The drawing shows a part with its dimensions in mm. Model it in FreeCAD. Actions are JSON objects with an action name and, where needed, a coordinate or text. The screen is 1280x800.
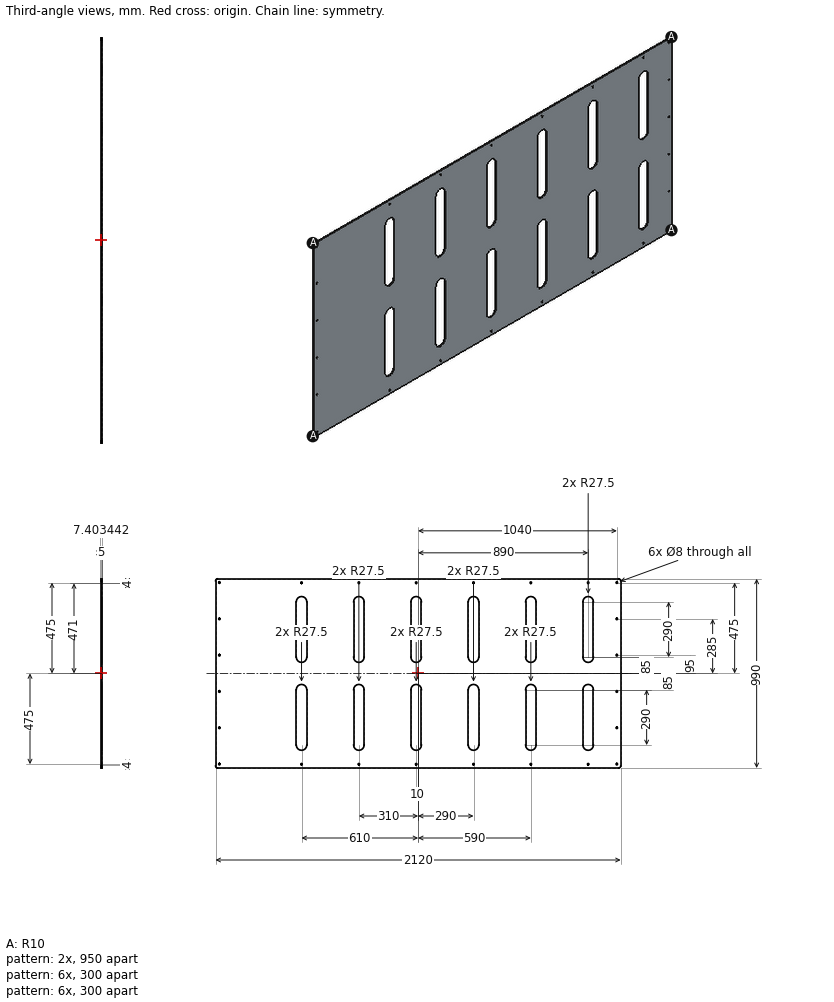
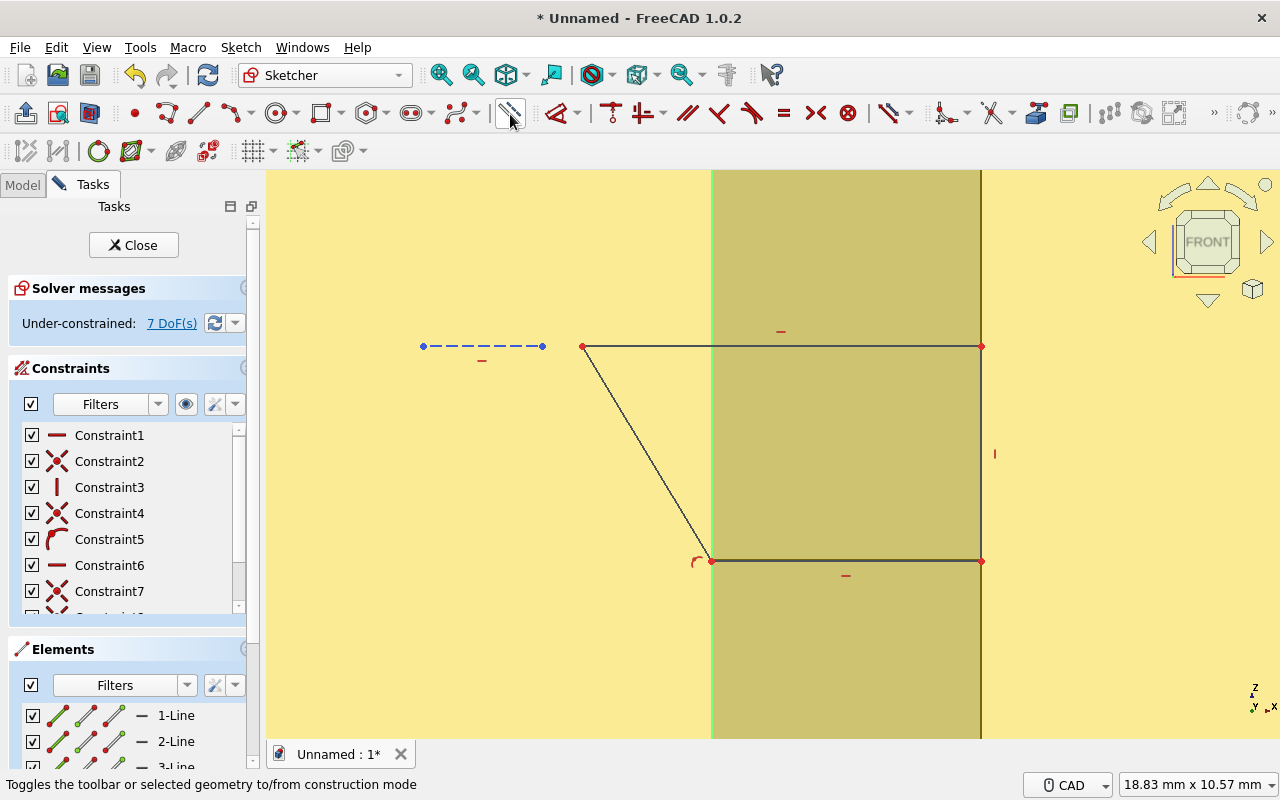
{"action": "left_click", "coordinate": [556, 114]}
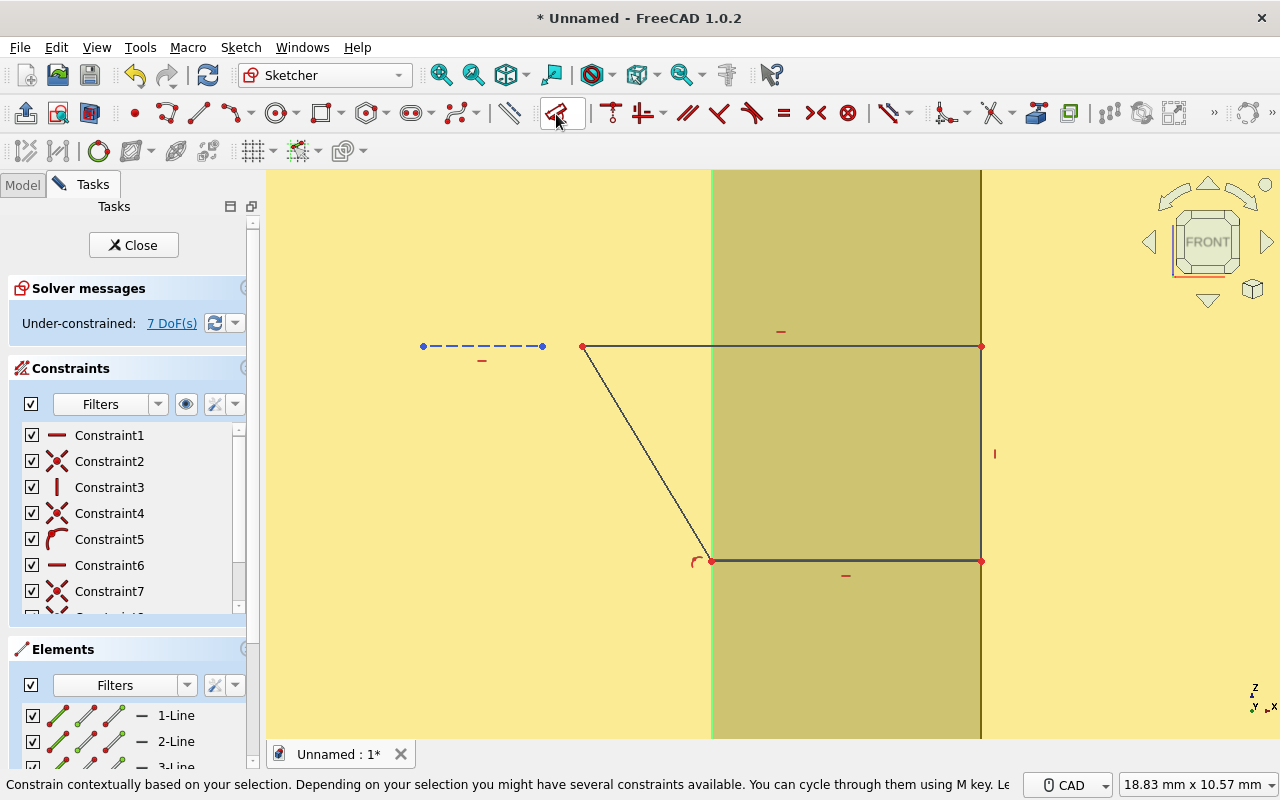
{"action": "left_click", "coordinate": [981, 411]}
{"action": "left_click", "coordinate": [1015, 454]}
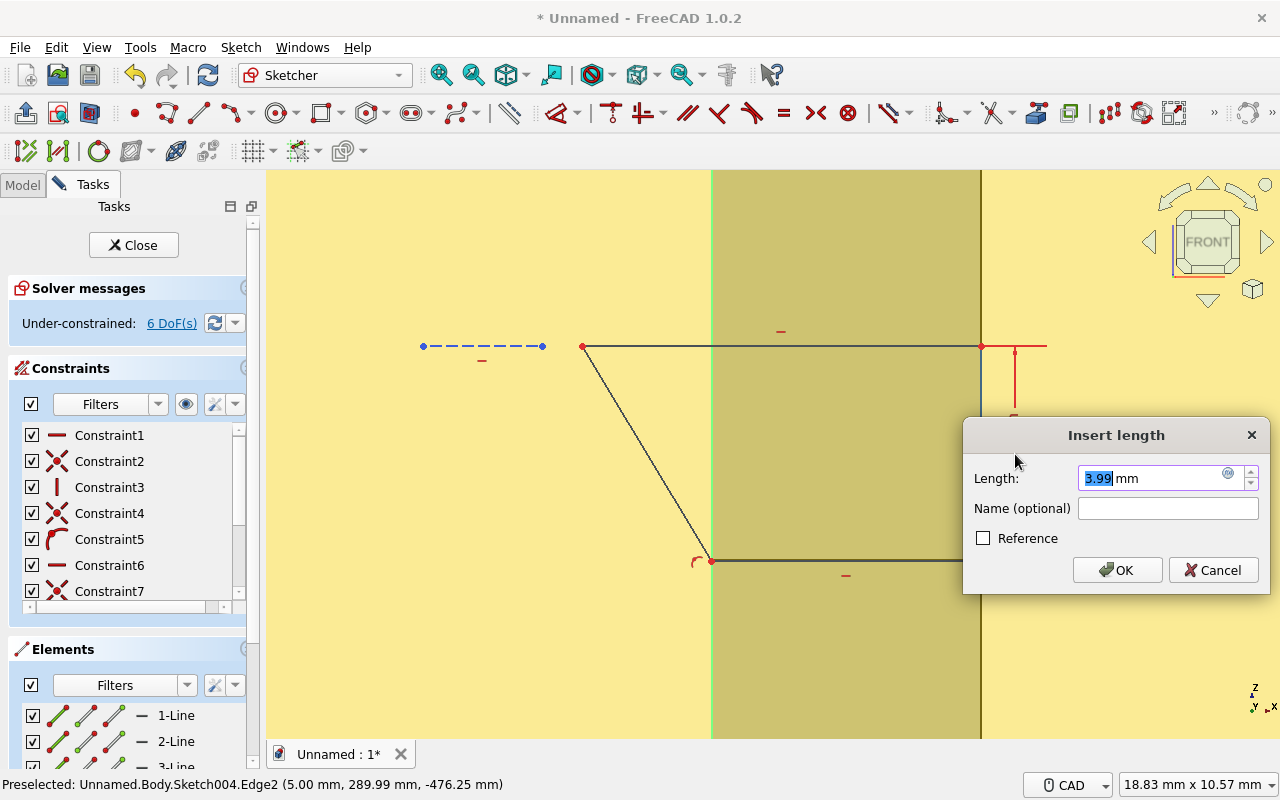
{"action": "type", "text": "4"}
{"action": "key", "text": "Return"}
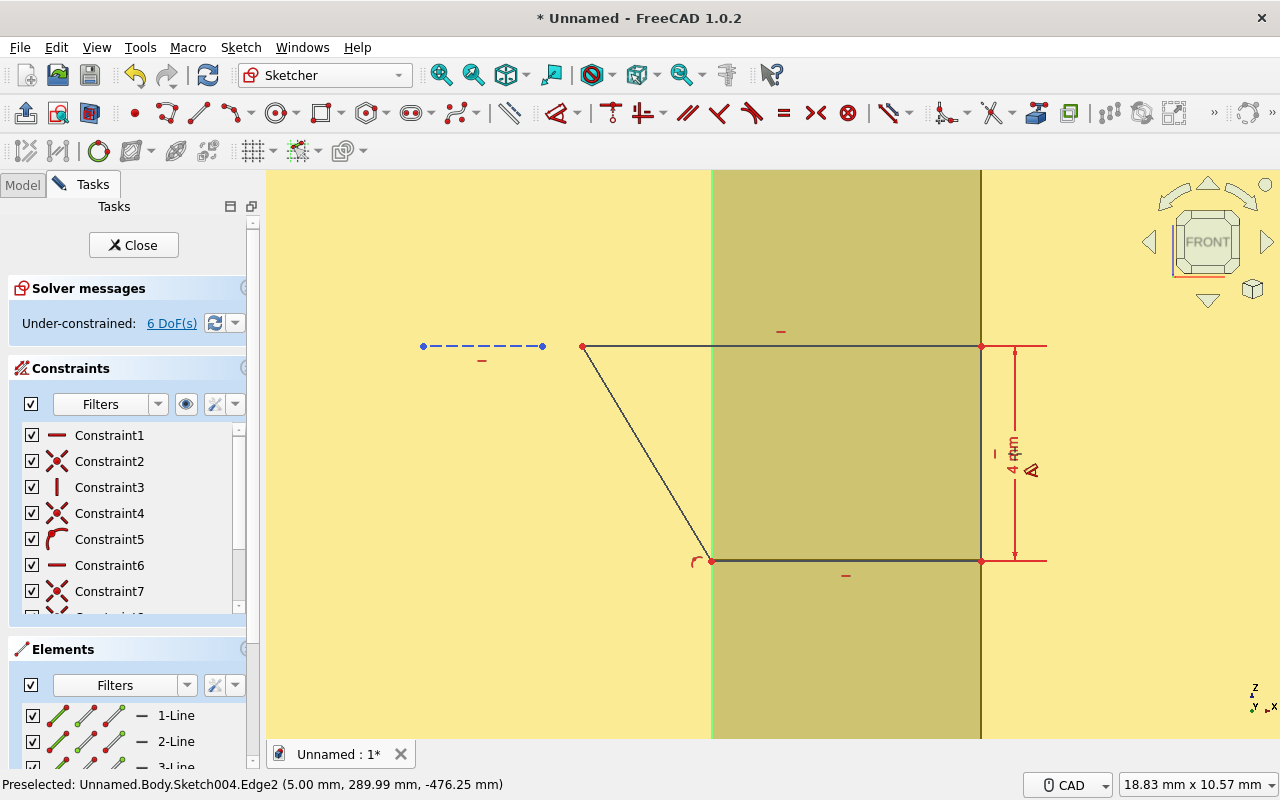
{"action": "left_click", "coordinate": [900, 561]}
{"action": "left_click", "coordinate": [846, 595]}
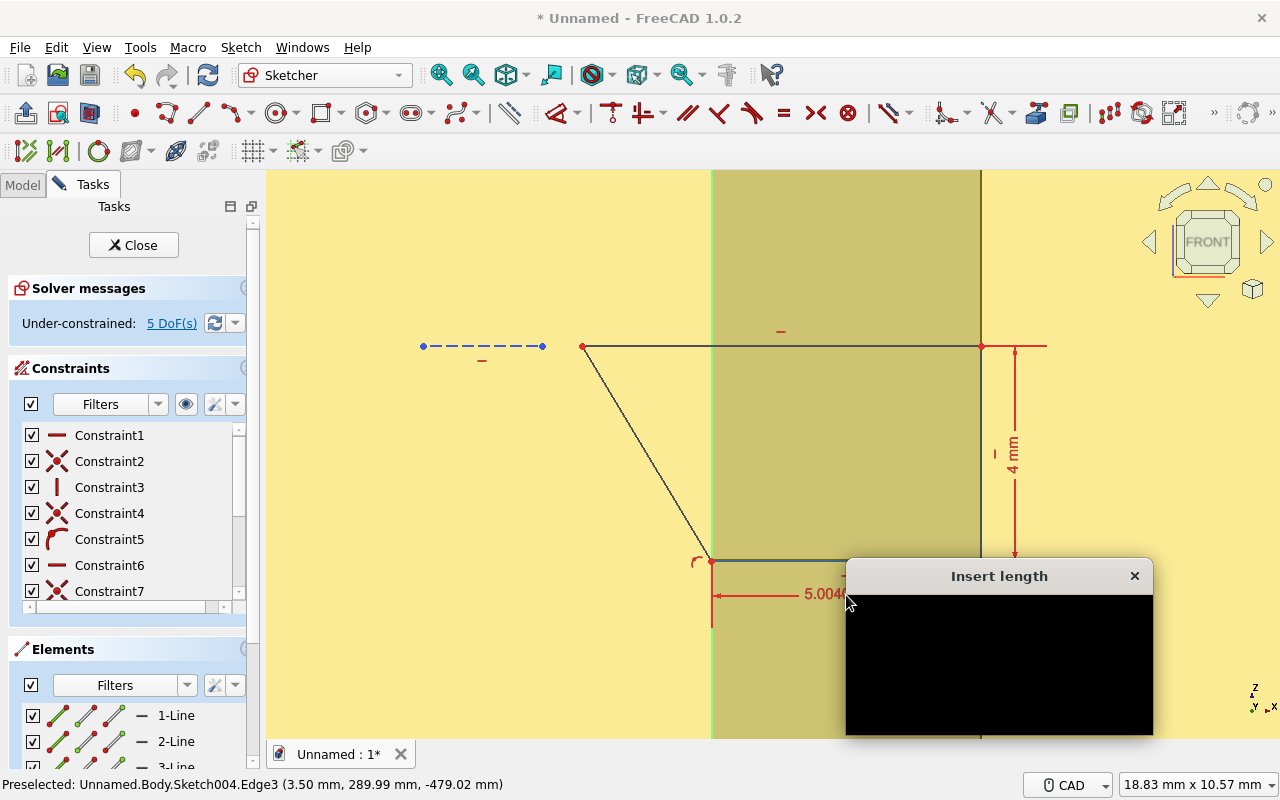
{"action": "type", "text": "5"}
{"action": "key", "text": "Return"}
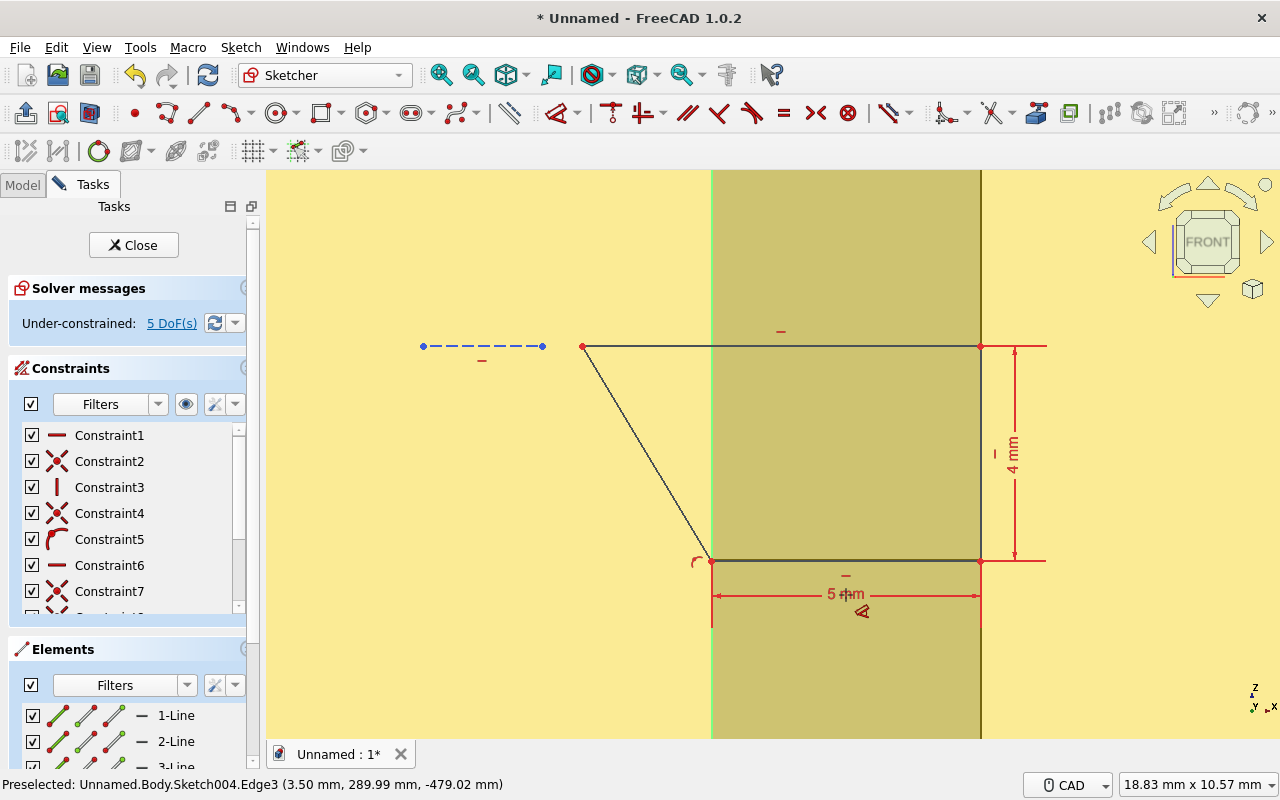
{"action": "left_click", "coordinate": [582, 346]}
{"action": "left_click", "coordinate": [548, 272]}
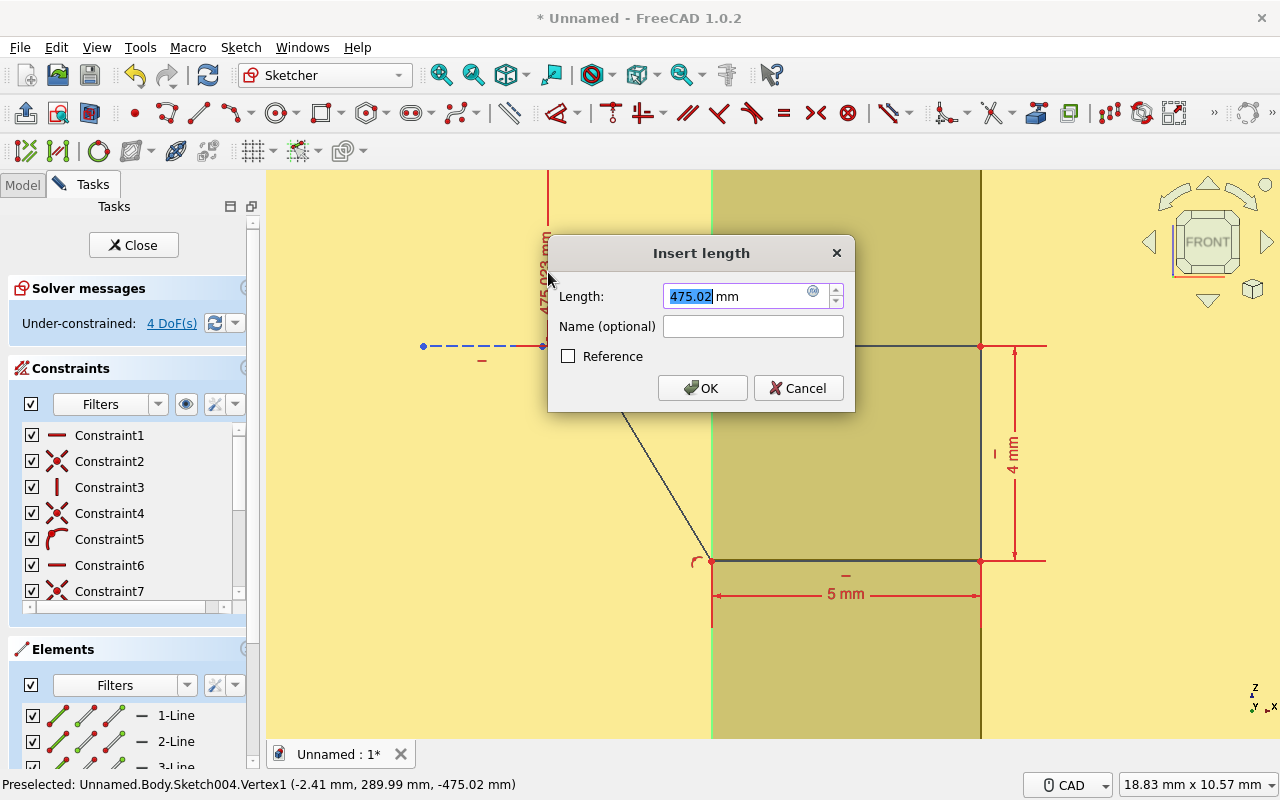
{"action": "type", "text": "475"}
{"action": "key", "text": "Return"}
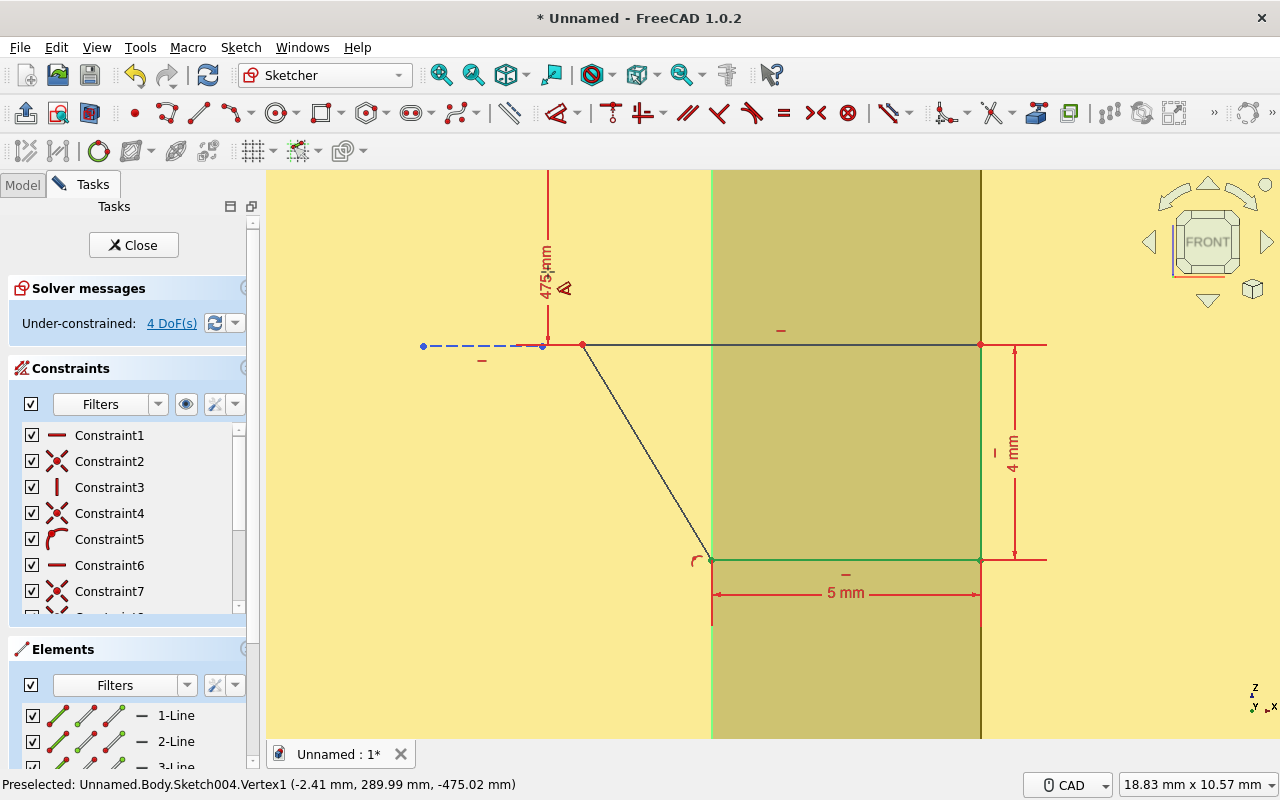
{"action": "left_click", "coordinate": [542, 346]}
{"action": "left_click", "coordinate": [508, 238]}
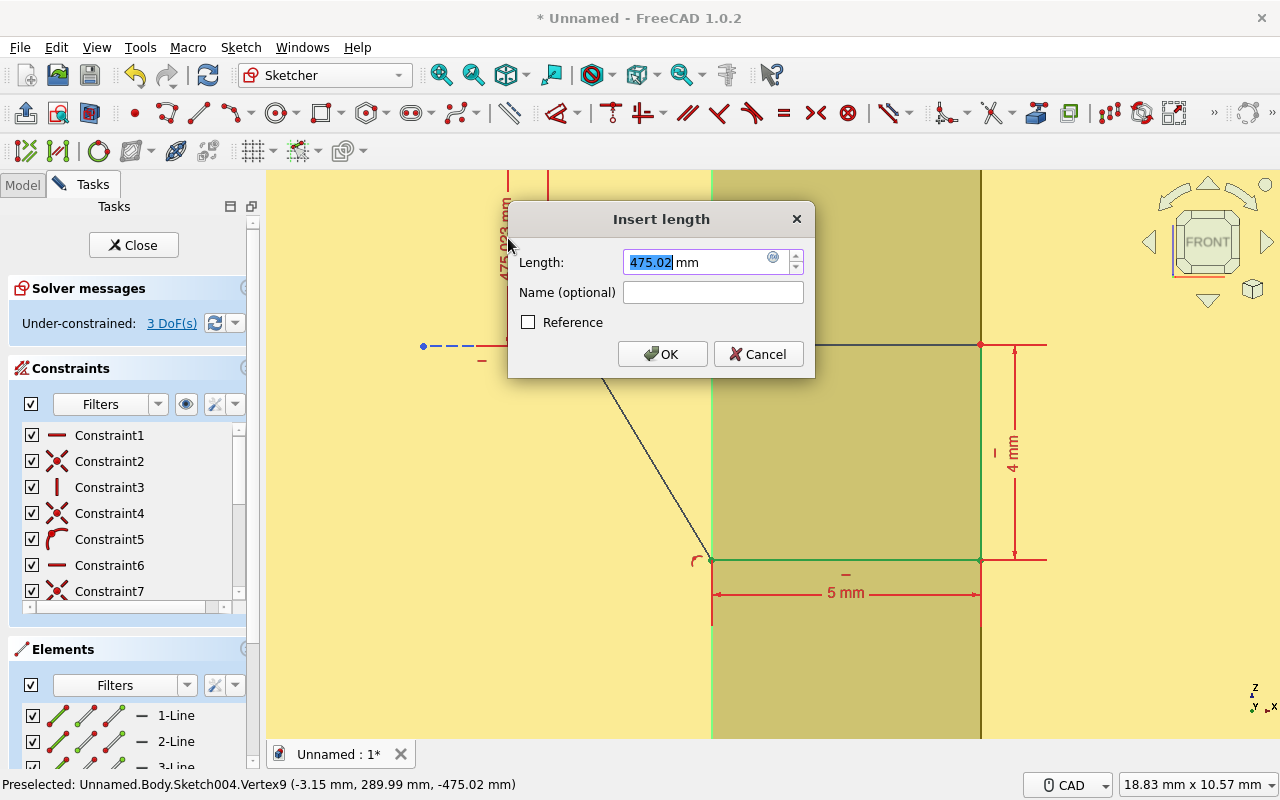
{"action": "type", "text": "475"}
{"action": "key", "text": "Return"}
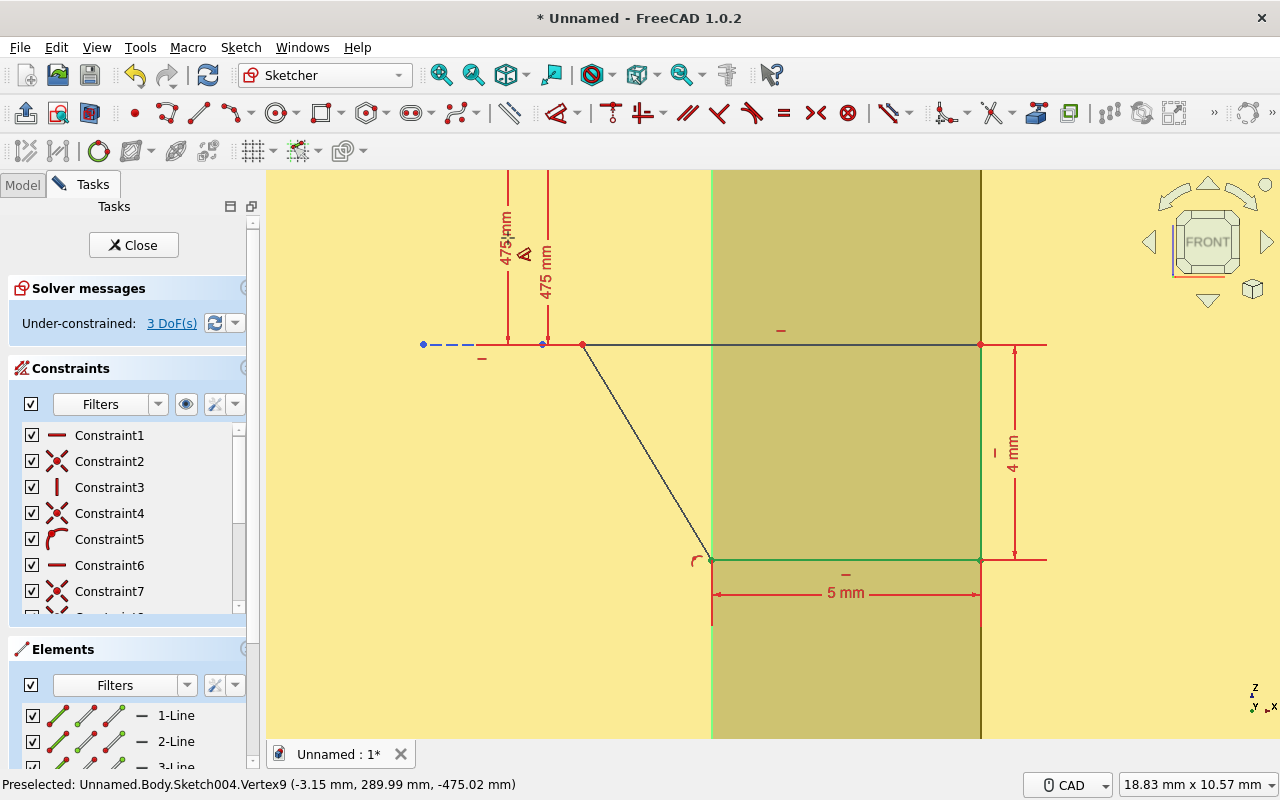
{"action": "scroll", "coordinate": [702, 345], "scroll_direction": "up", "scroll_amount": 2}